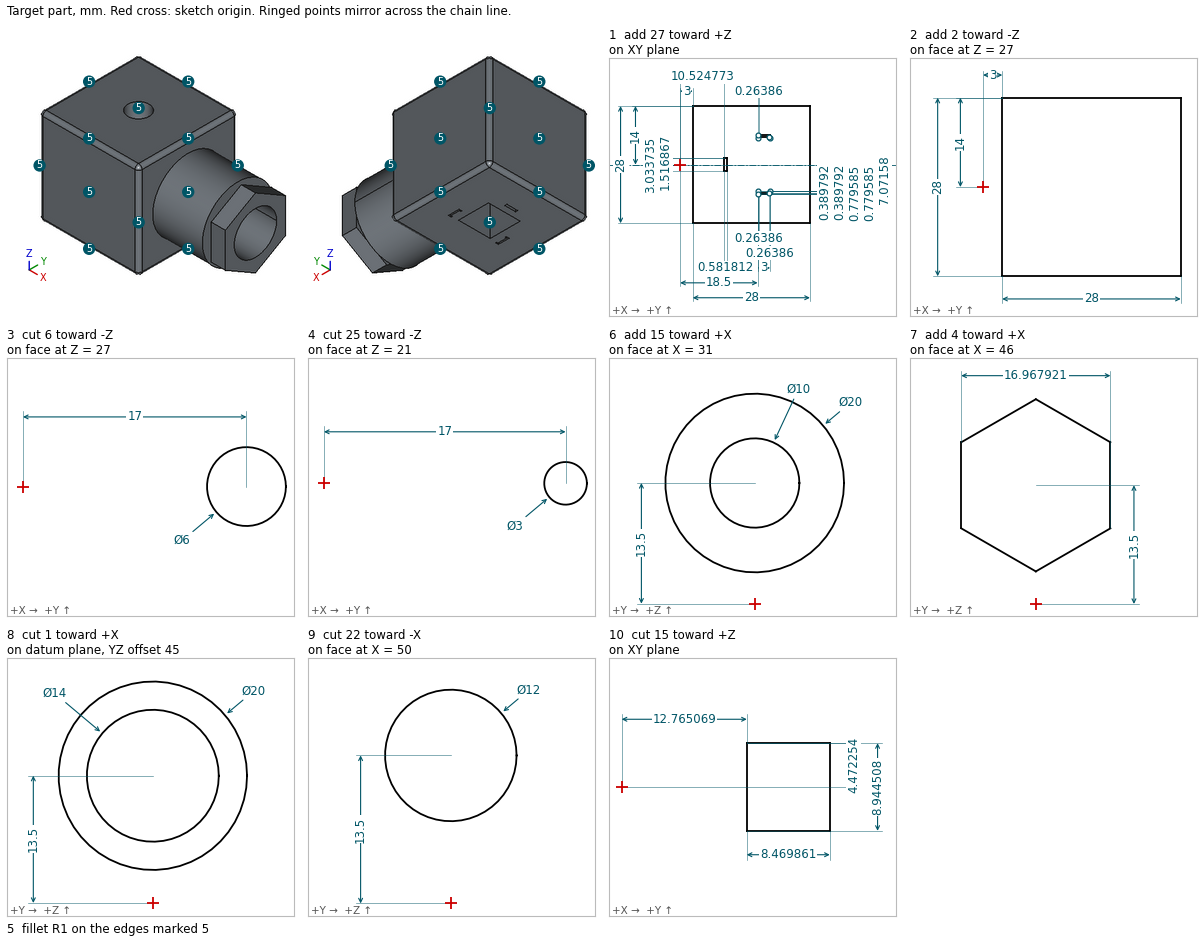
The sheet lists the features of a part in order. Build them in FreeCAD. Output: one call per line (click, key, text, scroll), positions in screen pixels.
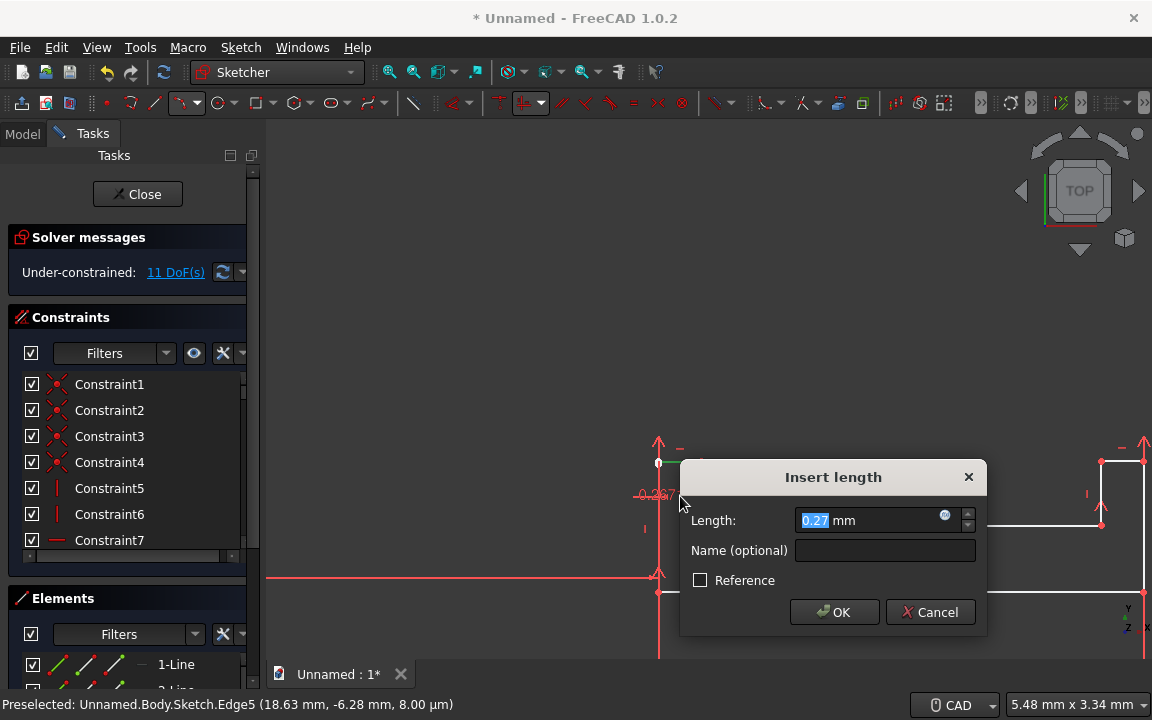
text(0.26386)
key(Return)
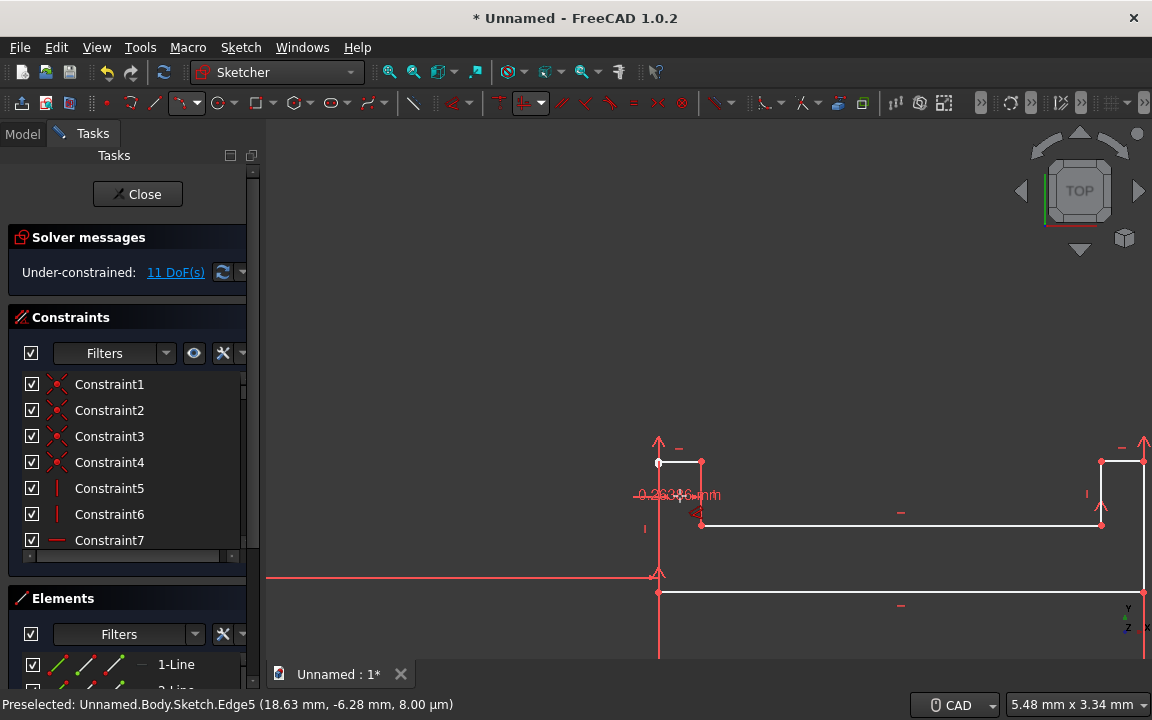
scroll(678, 465, down, 13)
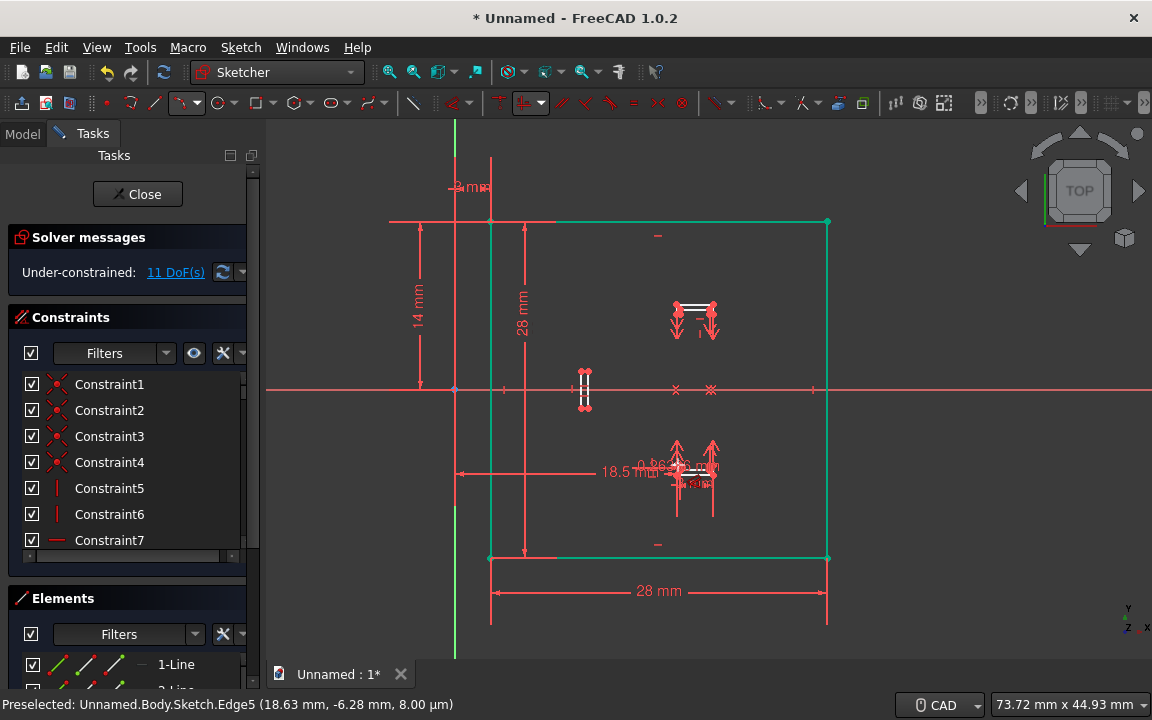
scroll(711, 465, up, 14)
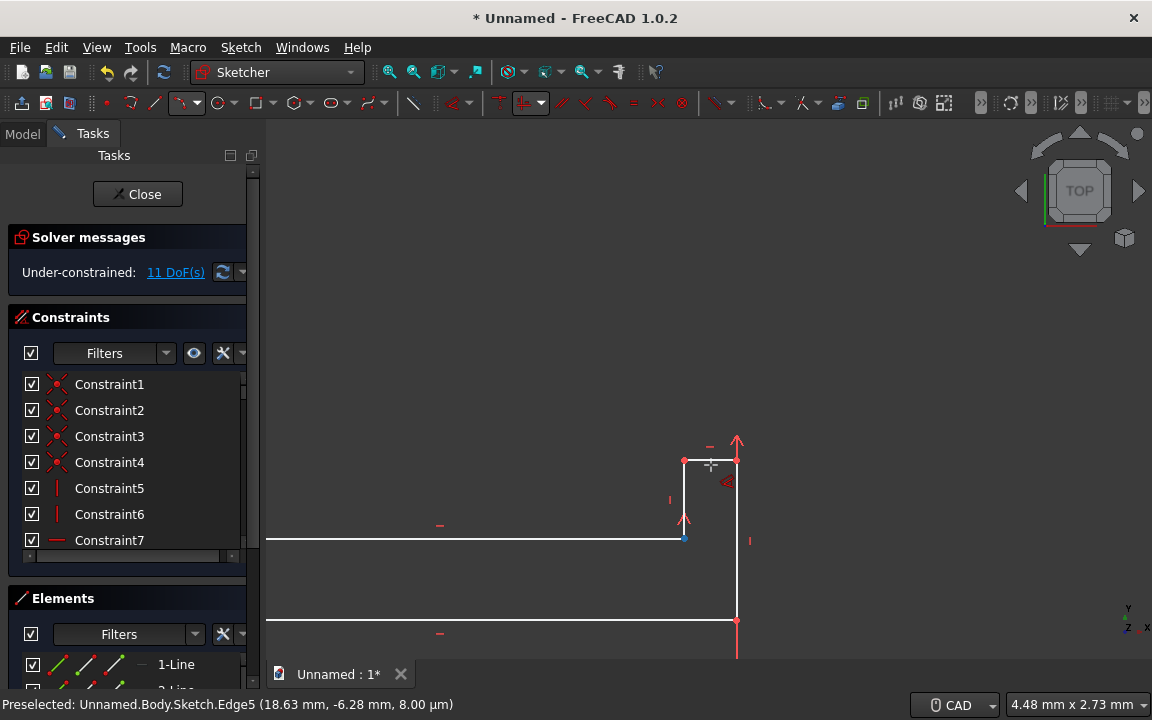
click(700, 460)
click(711, 494)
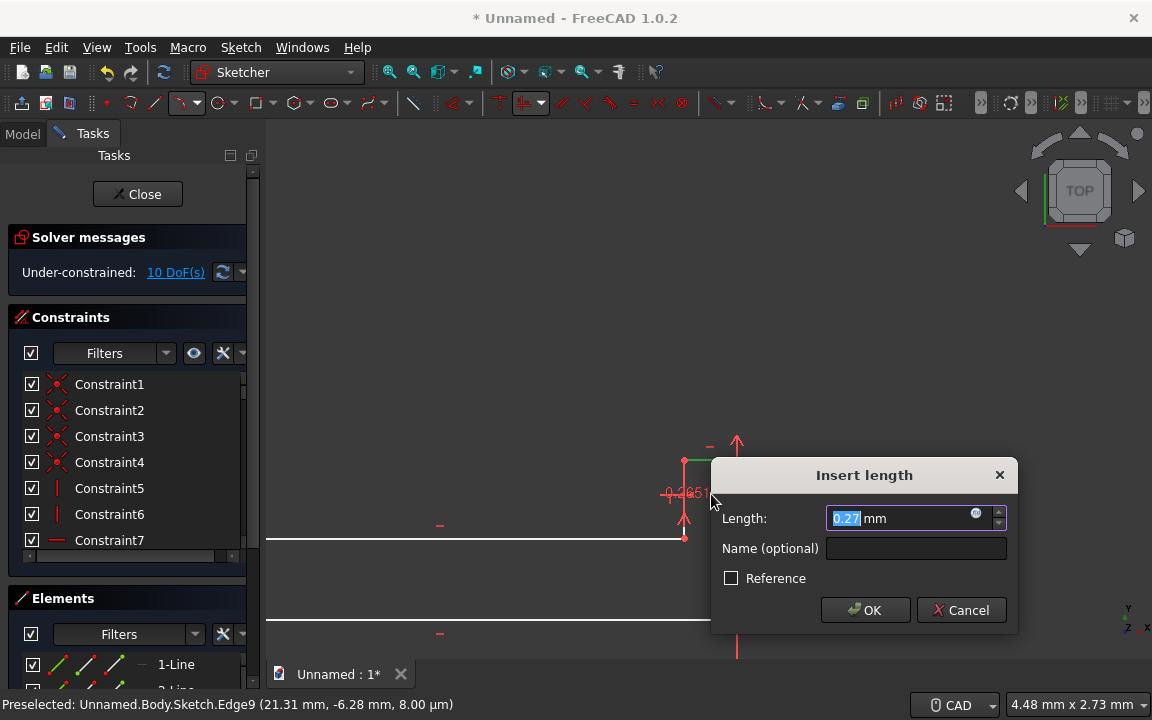
text(0.26386)
key(Return)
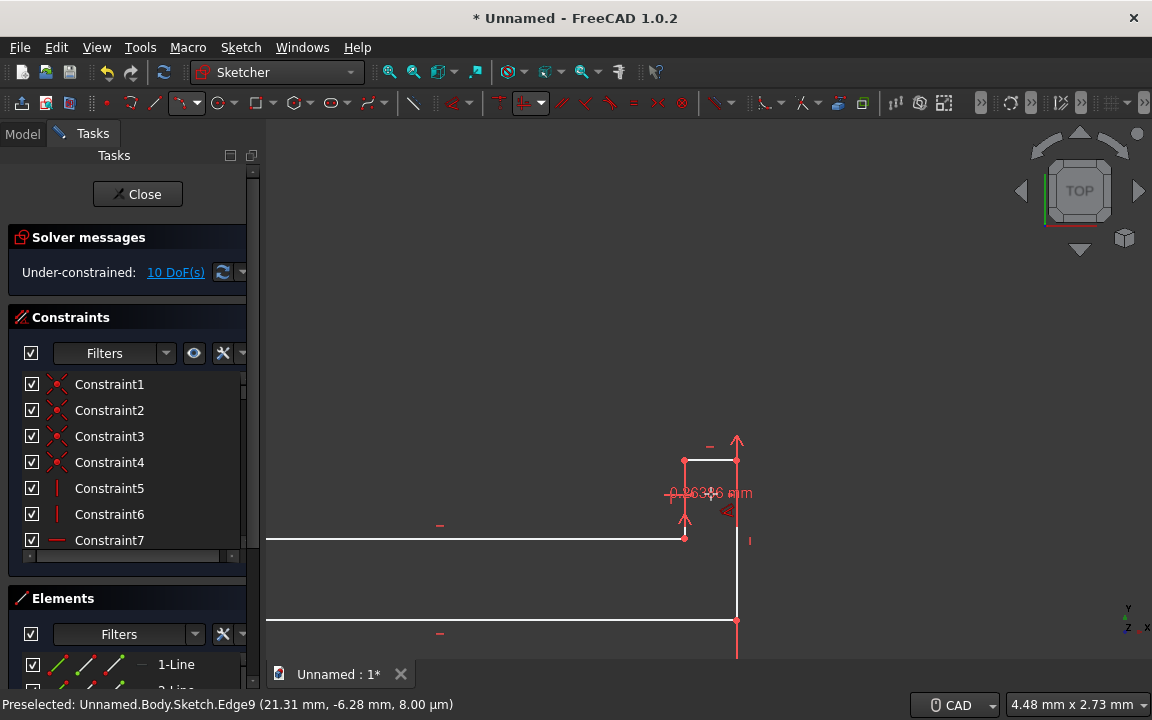
scroll(711, 465, down, 14)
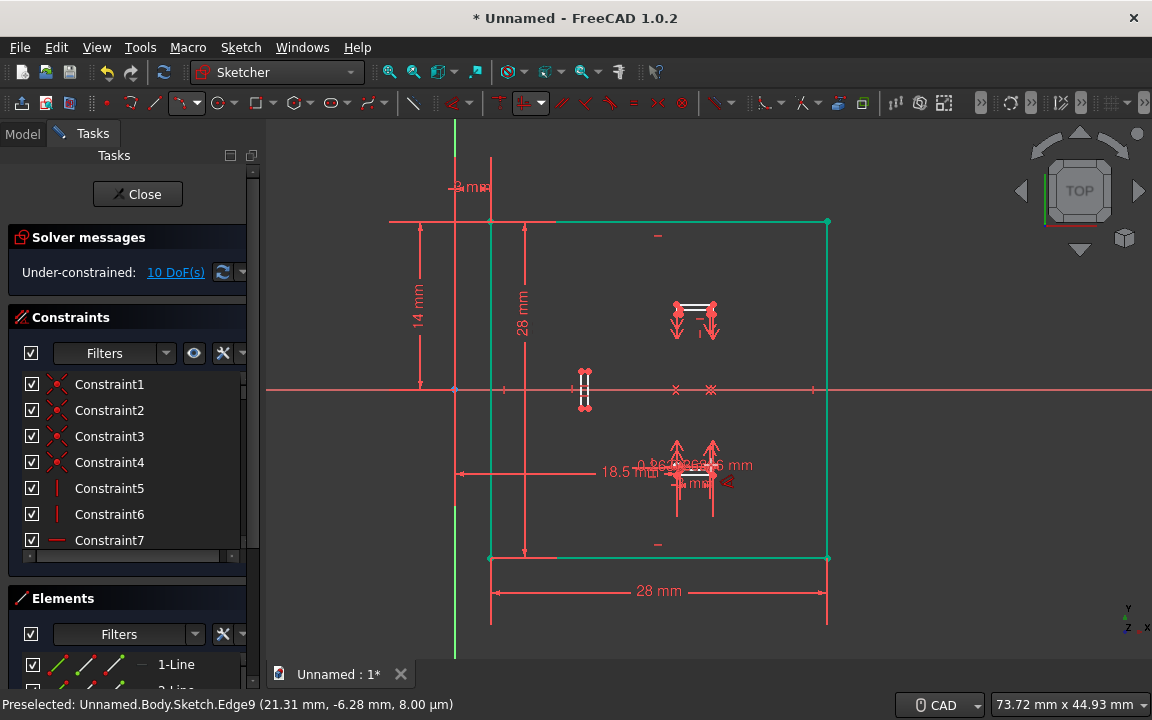
scroll(679, 314, up, 14)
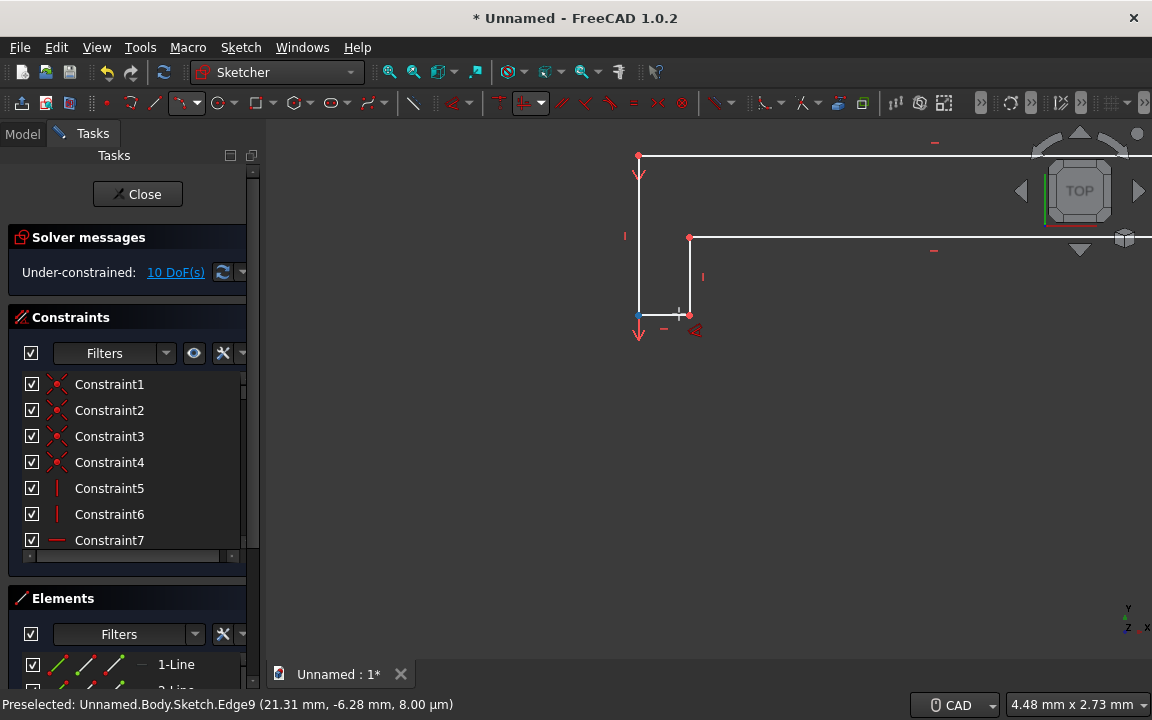
click(675, 315)
click(664, 281)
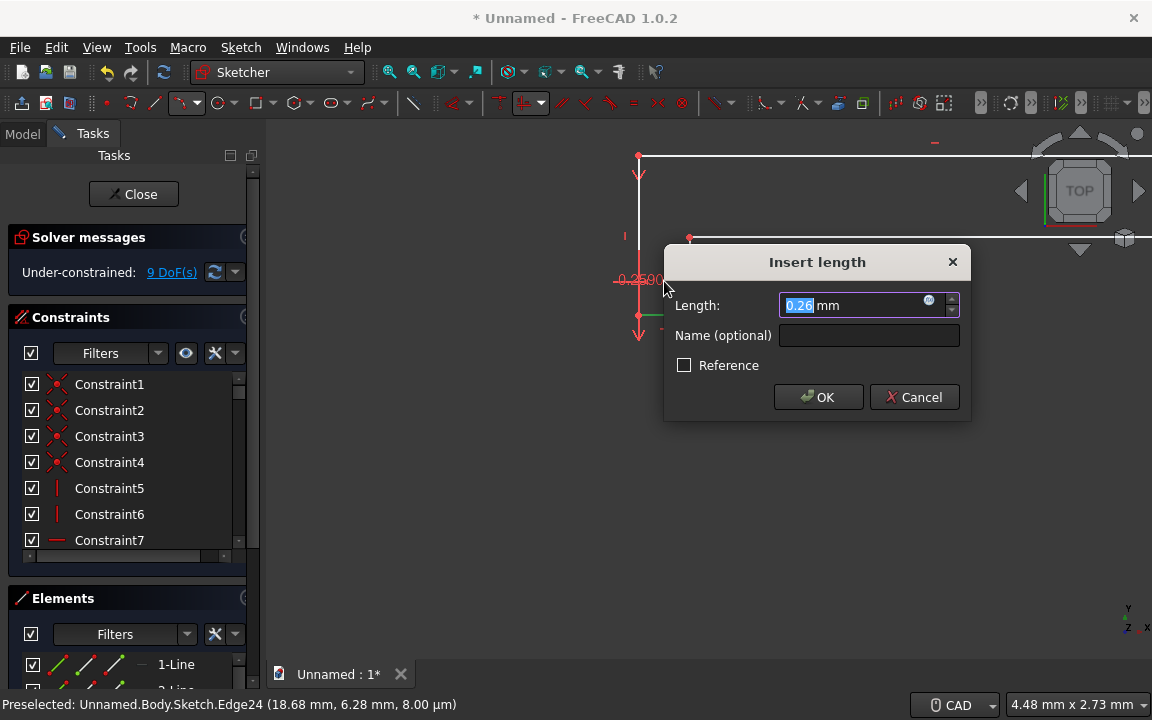
text(0.26386)
key(Return)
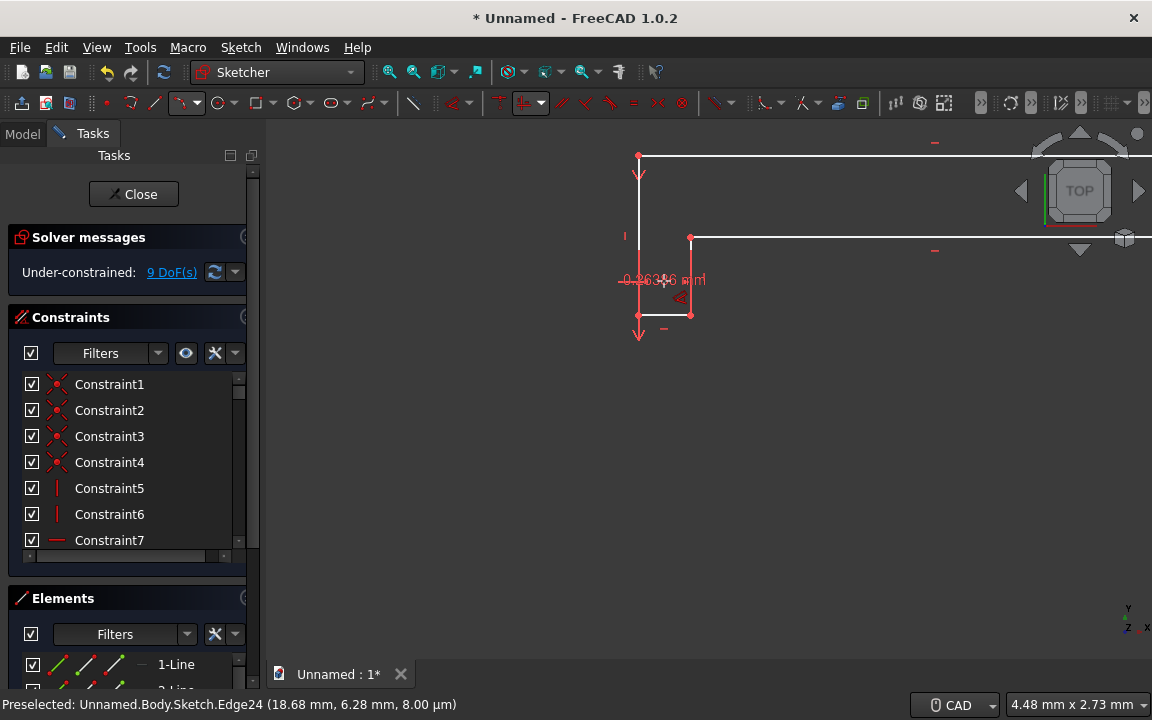
scroll(679, 313, down, 14)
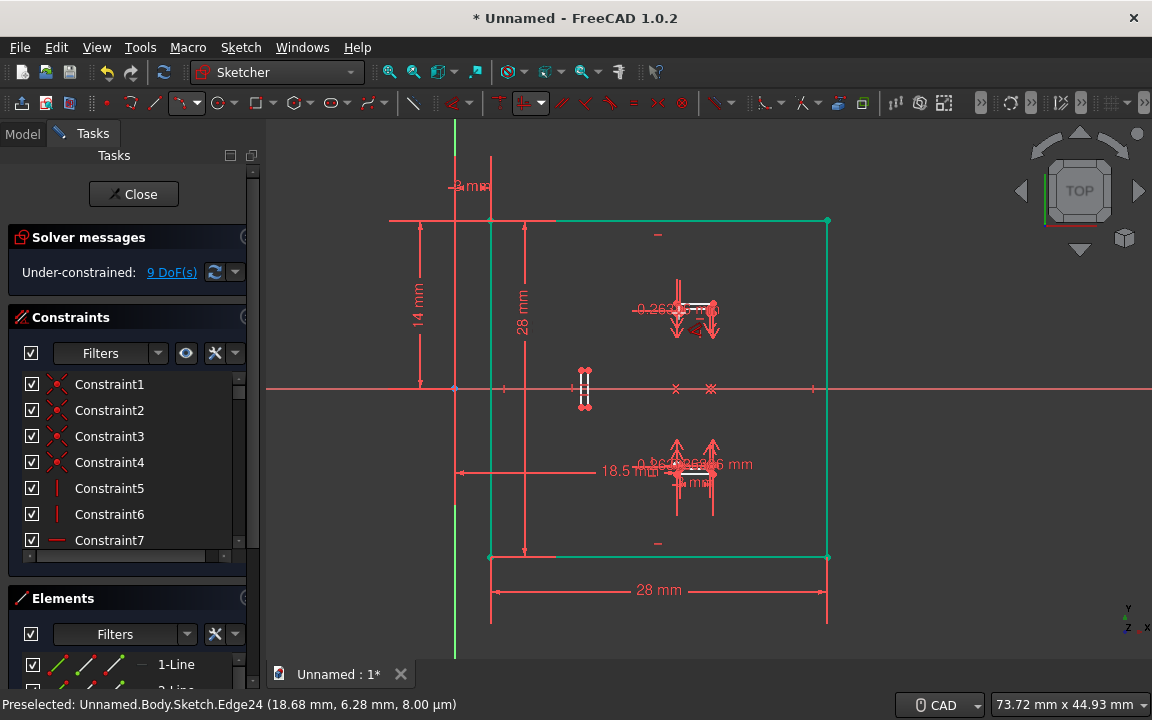
scroll(680, 466, up, 12)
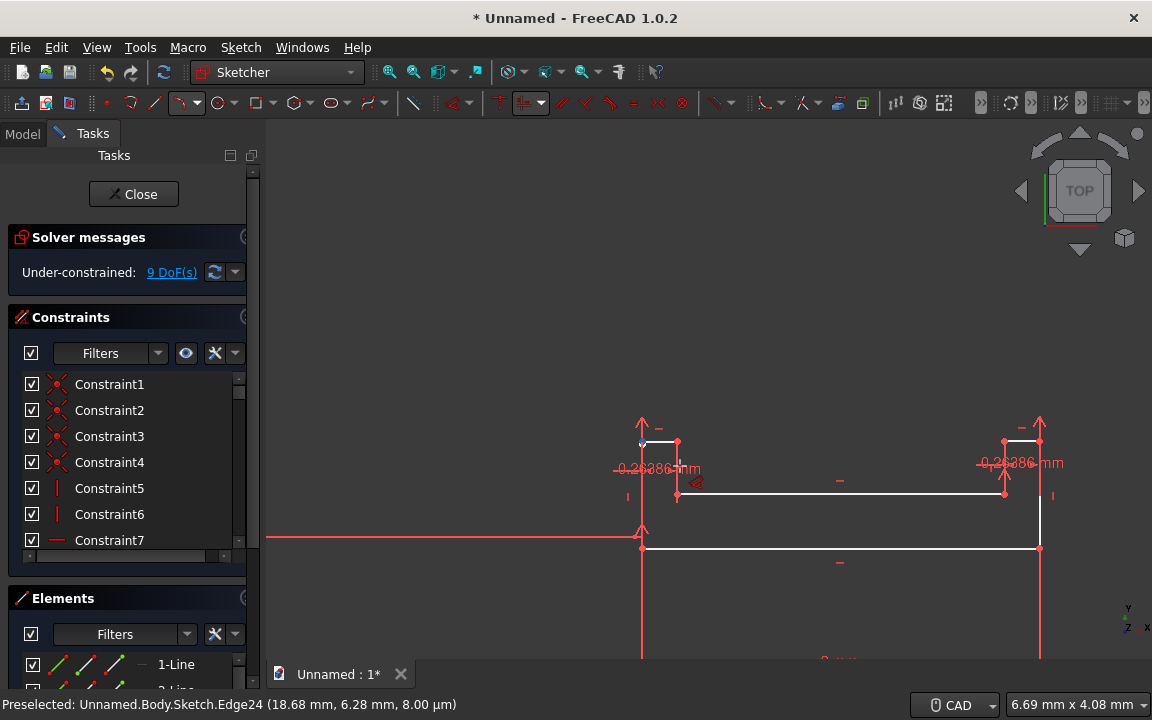
click(677, 458)
click(735, 468)